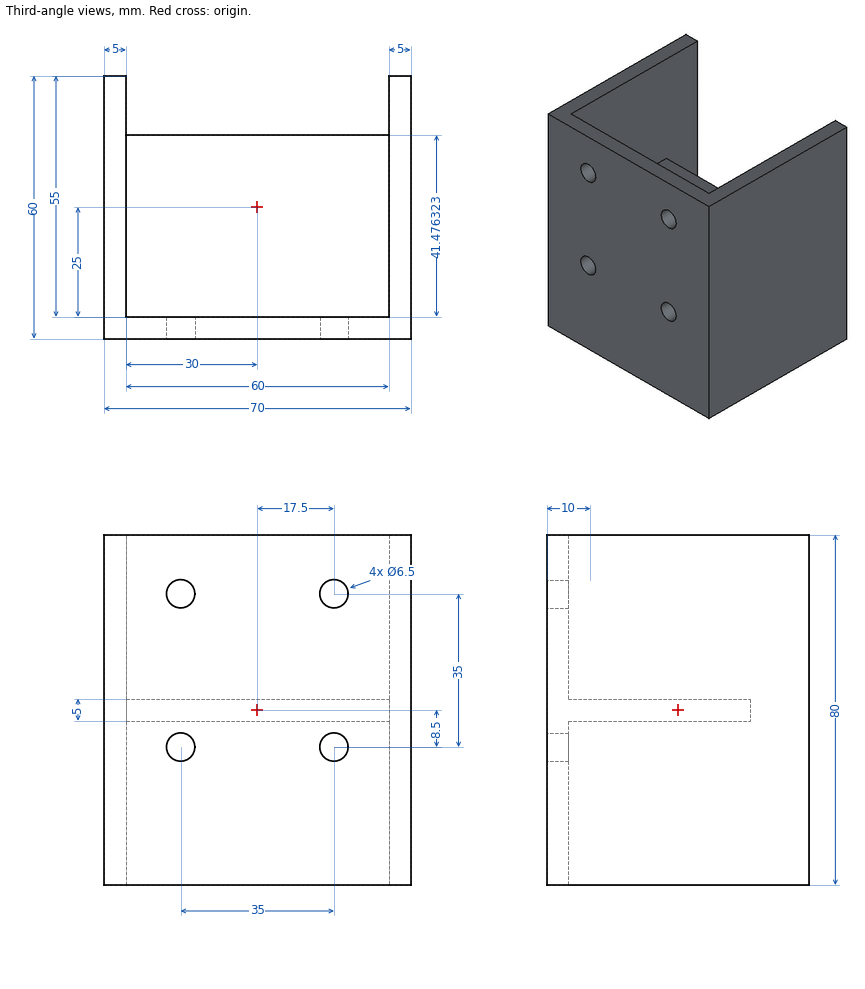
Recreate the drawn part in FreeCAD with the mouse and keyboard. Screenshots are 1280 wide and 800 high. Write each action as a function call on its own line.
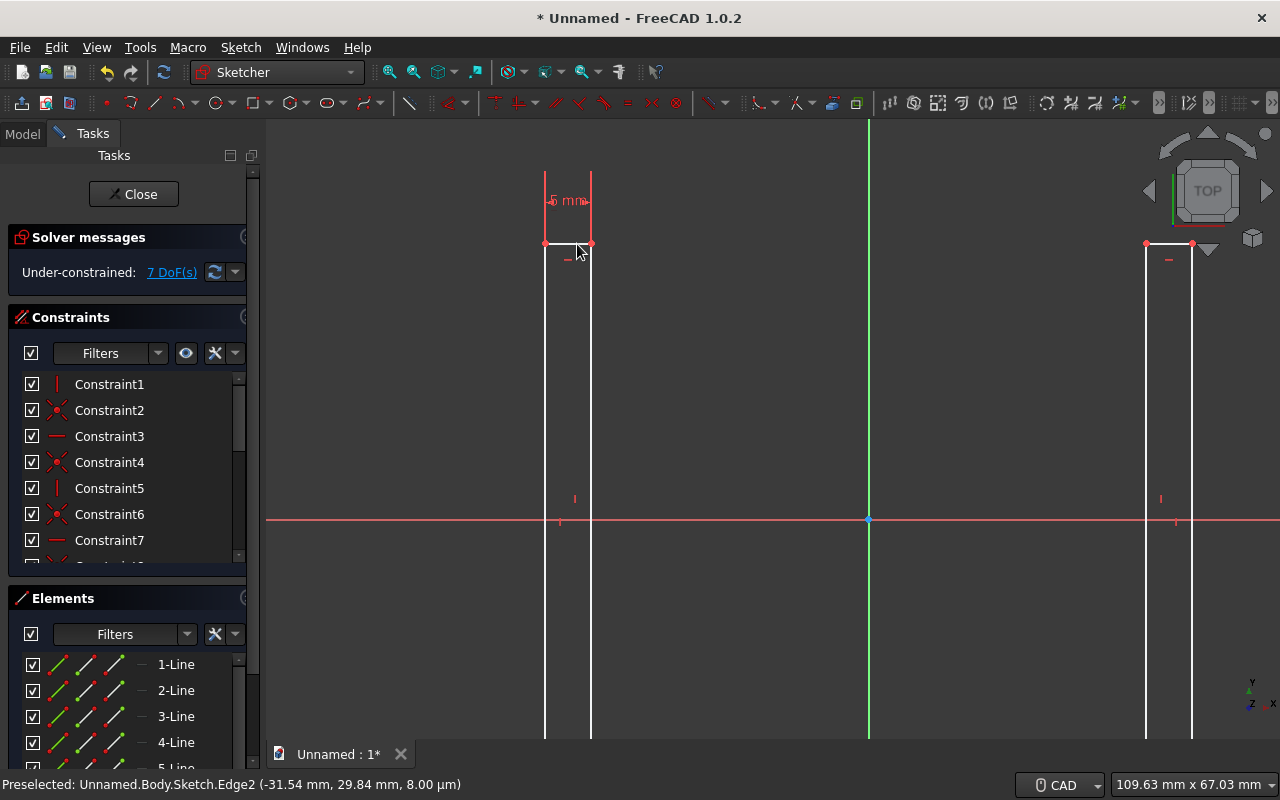
scroll(371, 244, down, 2)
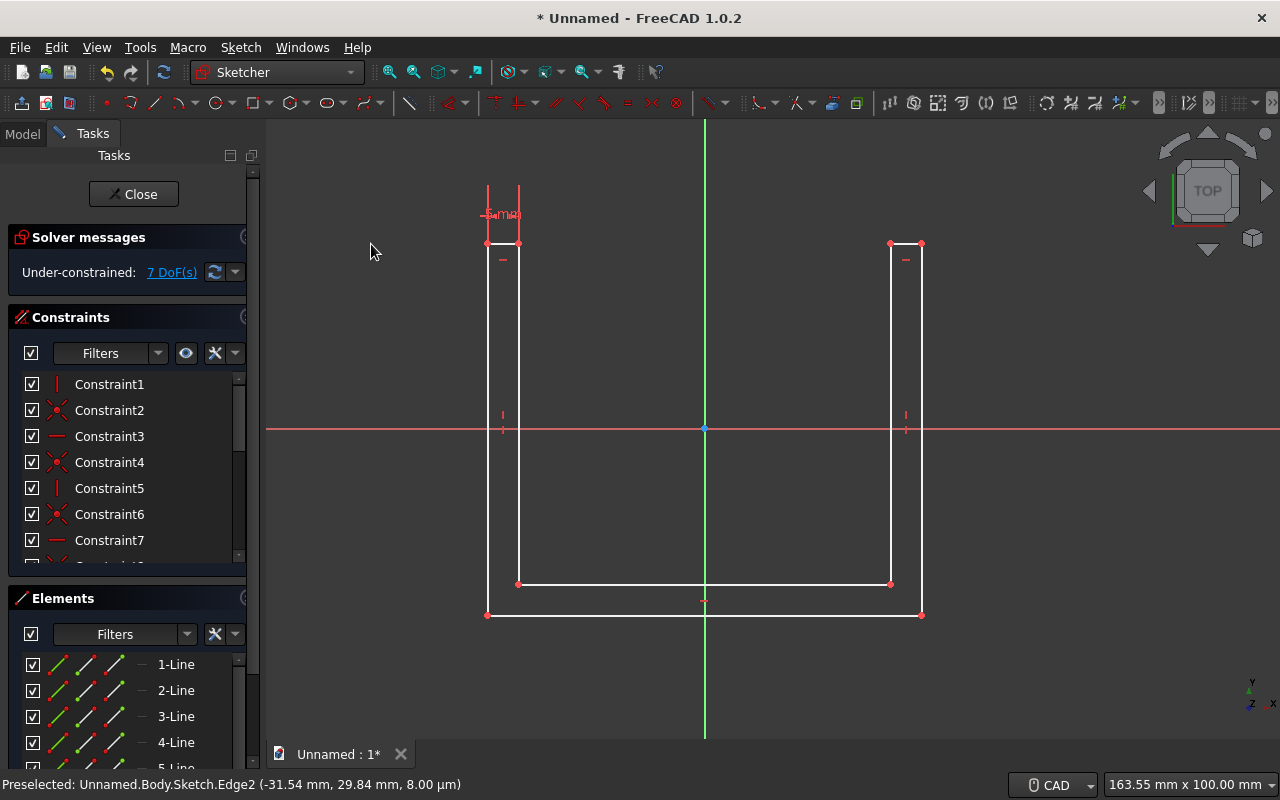
scroll(912, 244, up, 2)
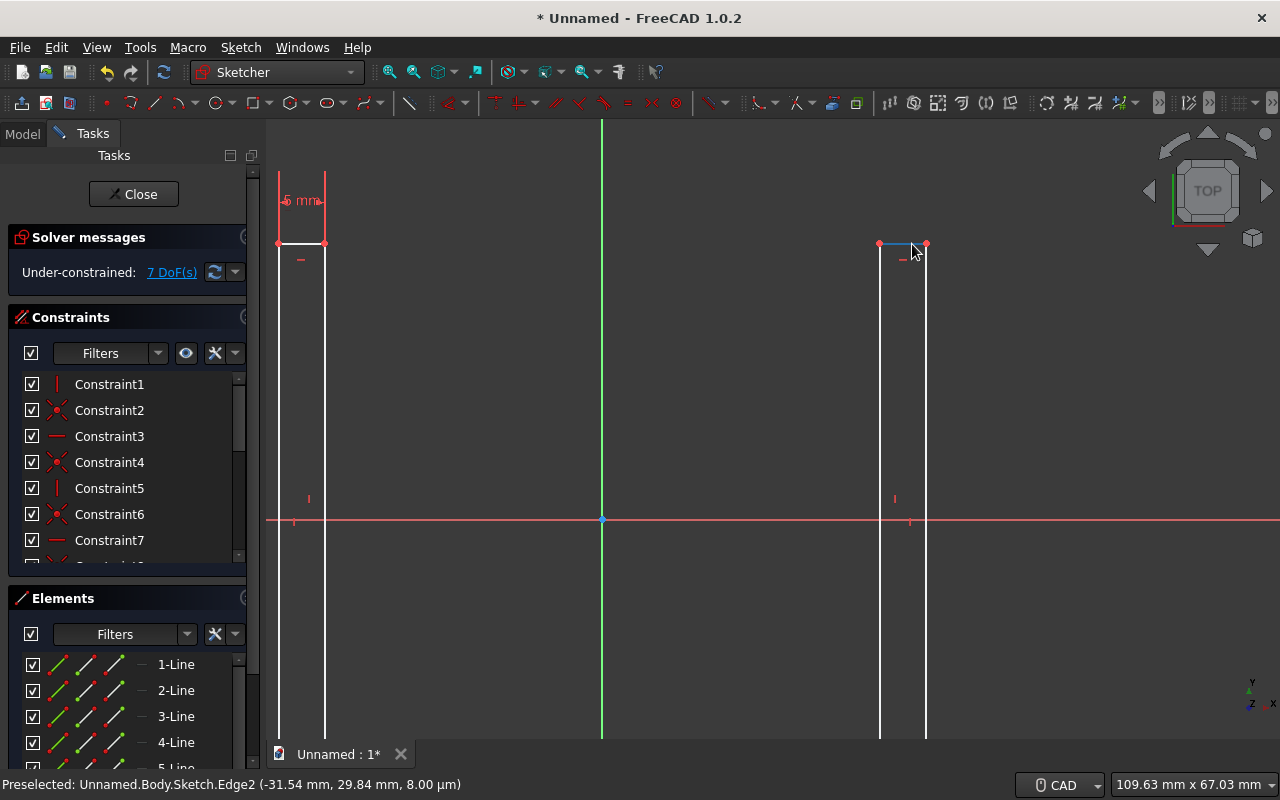
click(912, 244)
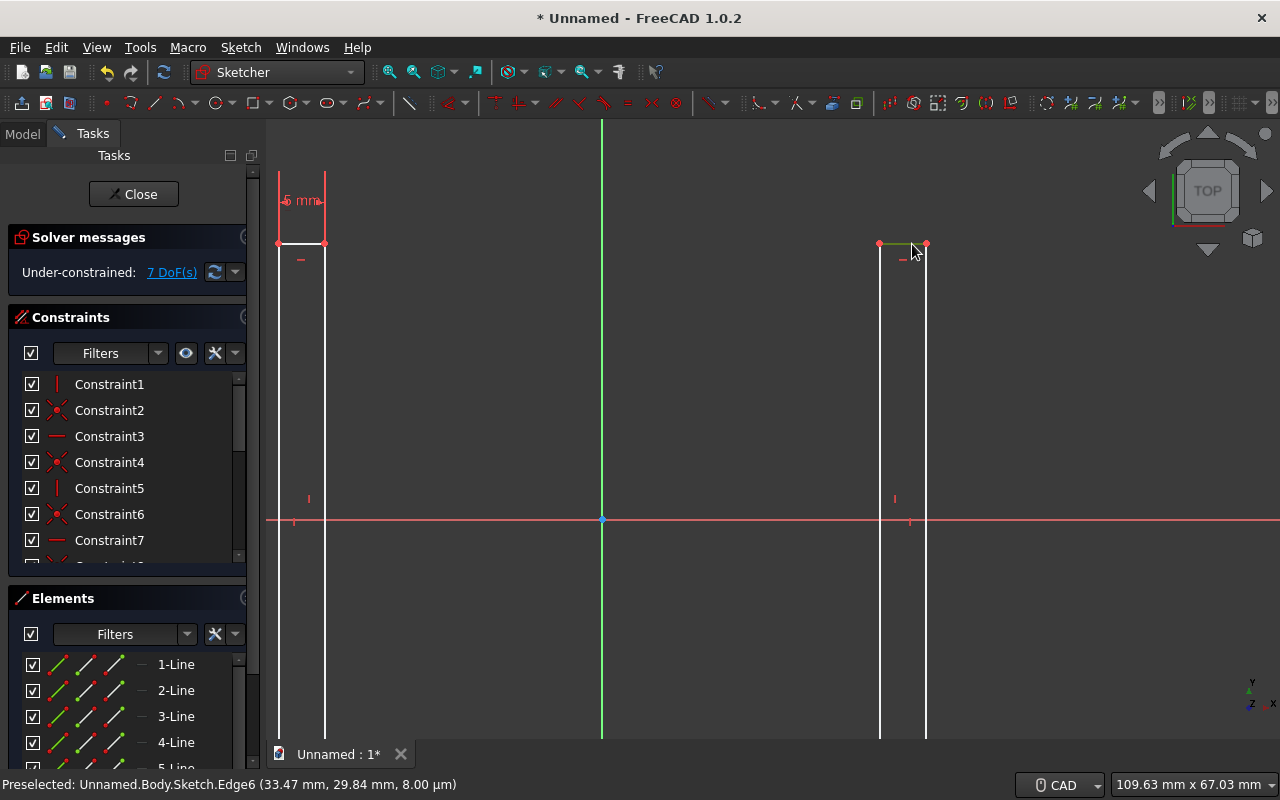
key(l)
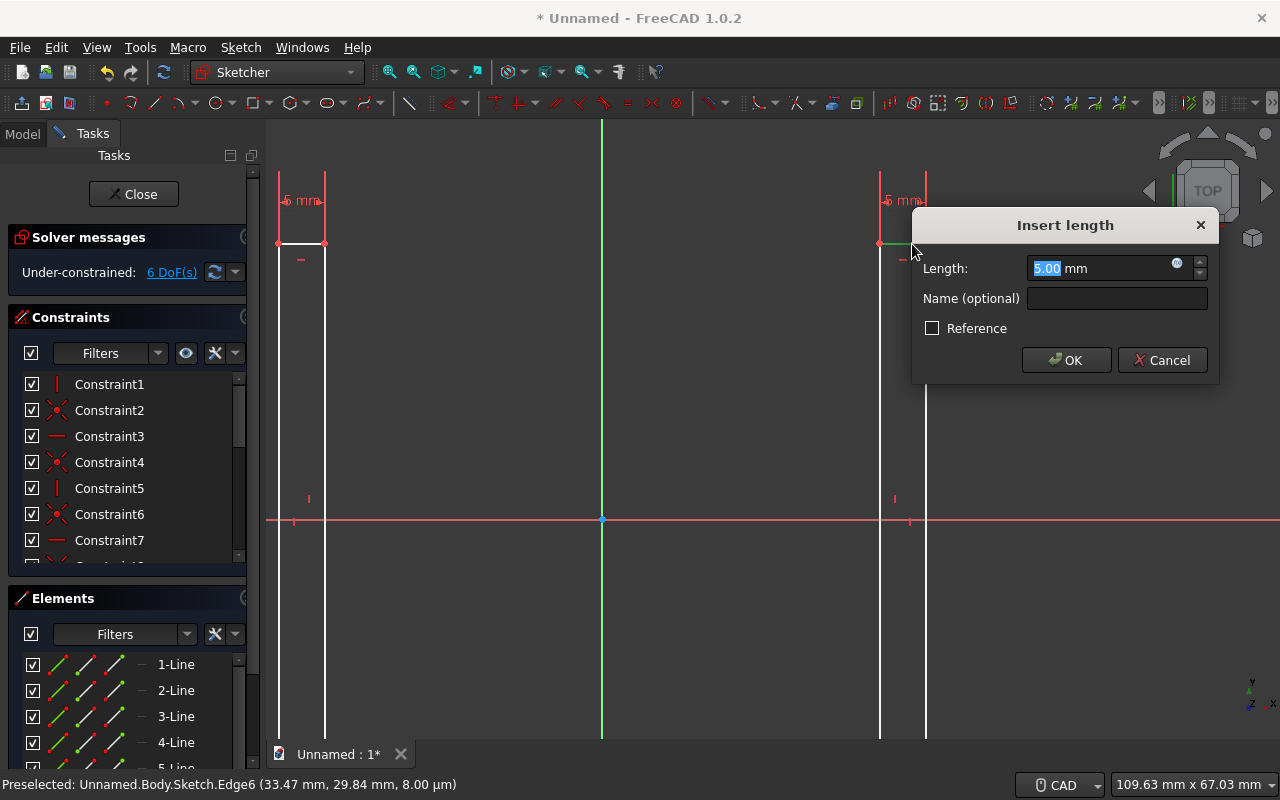
text(5)
key(Return)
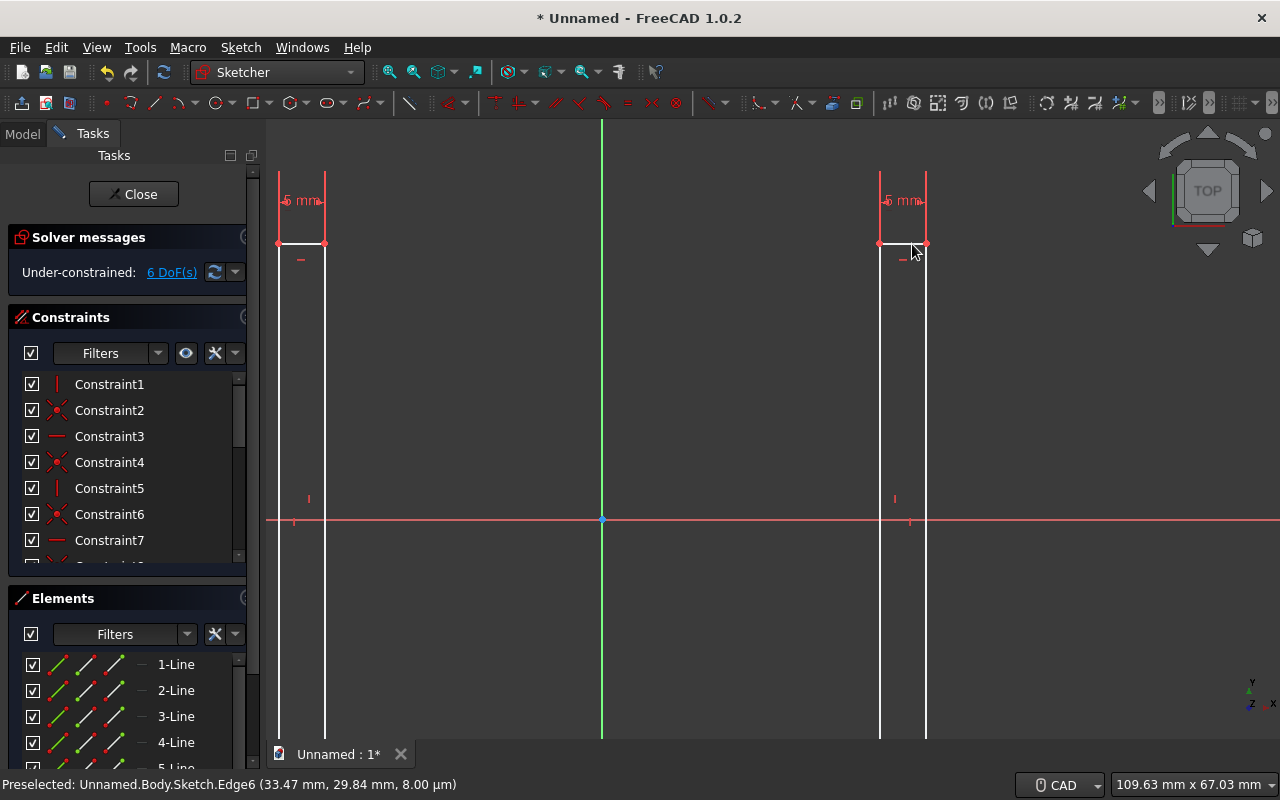
click(325, 600)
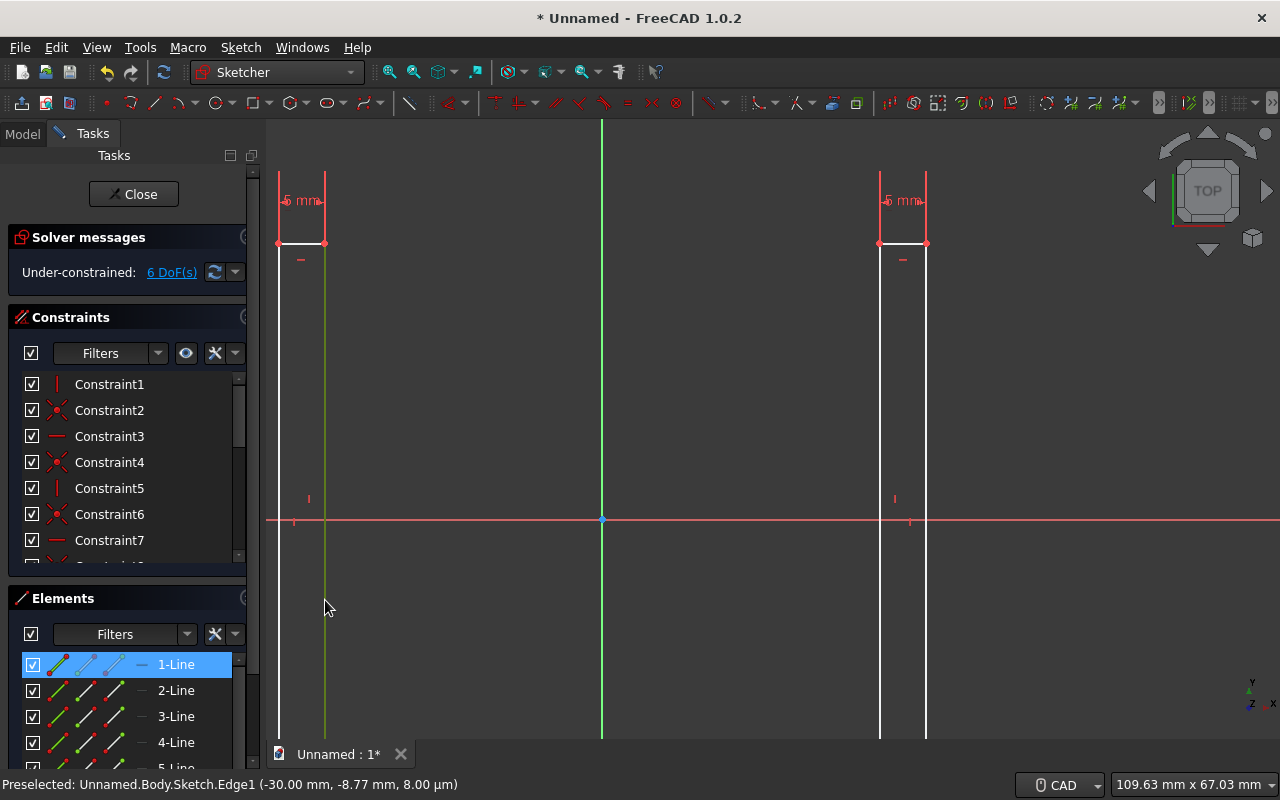
key(i)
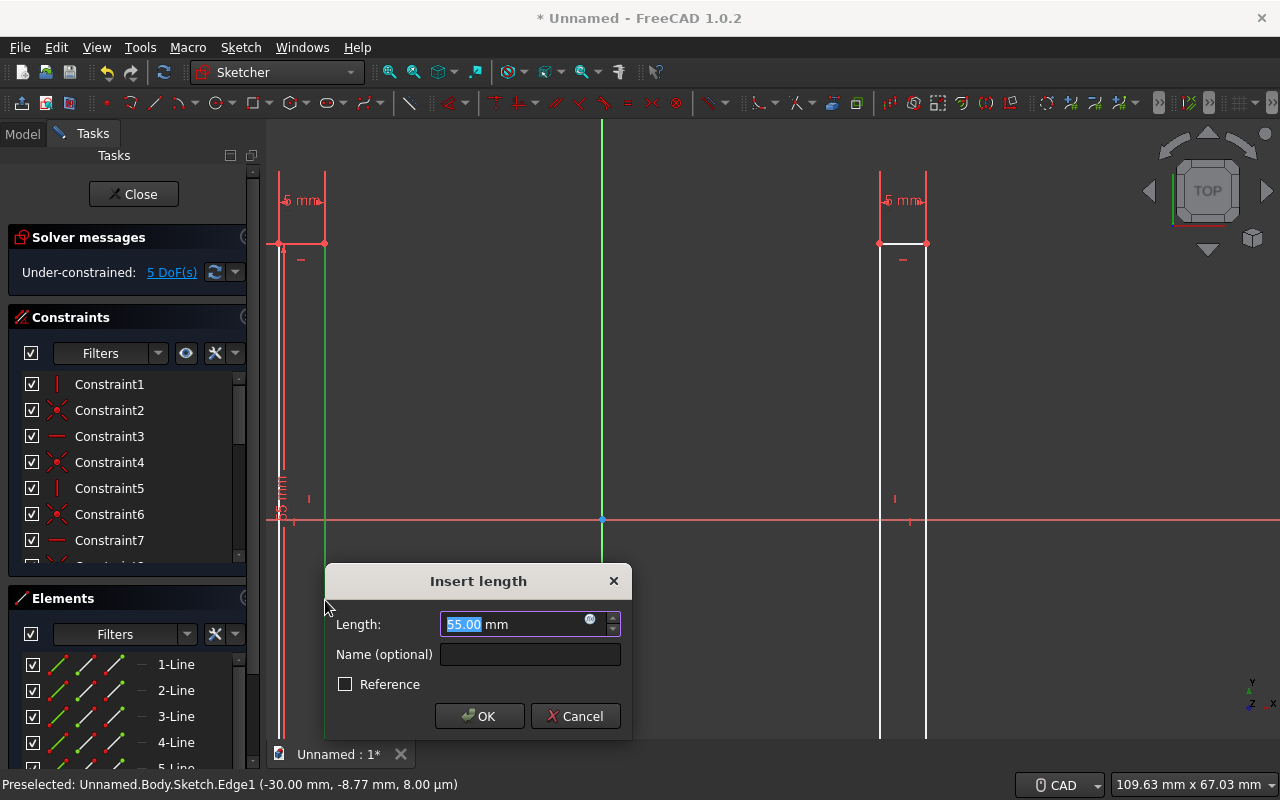
text(55)
key(Return)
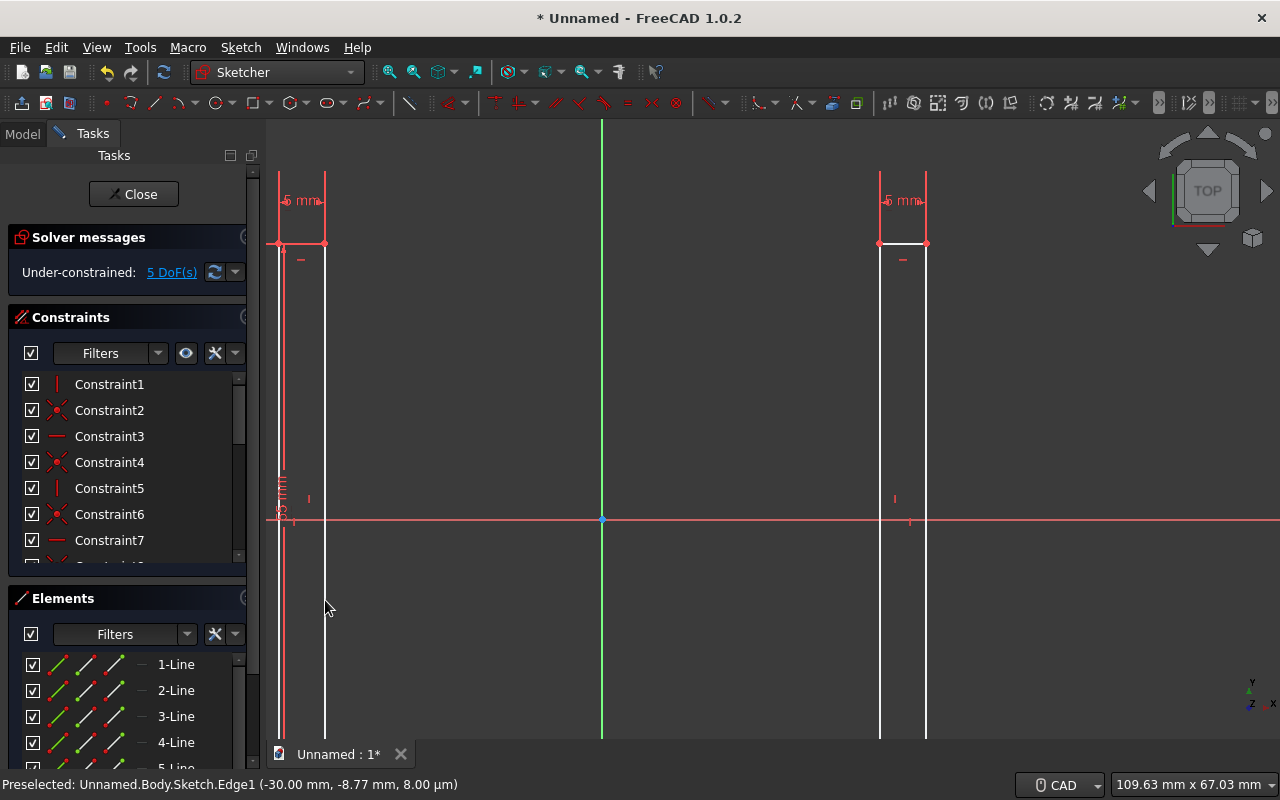
scroll(912, 244, down, 2)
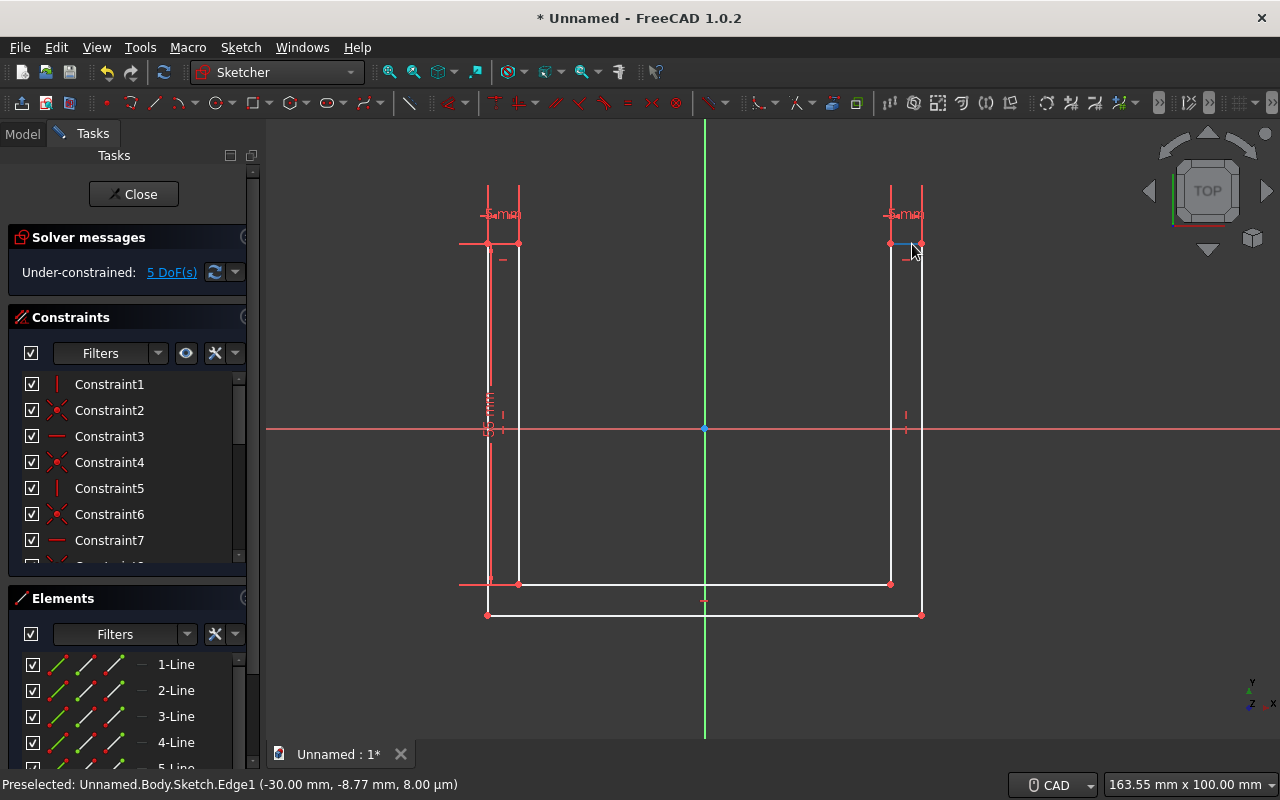
click(488, 356)